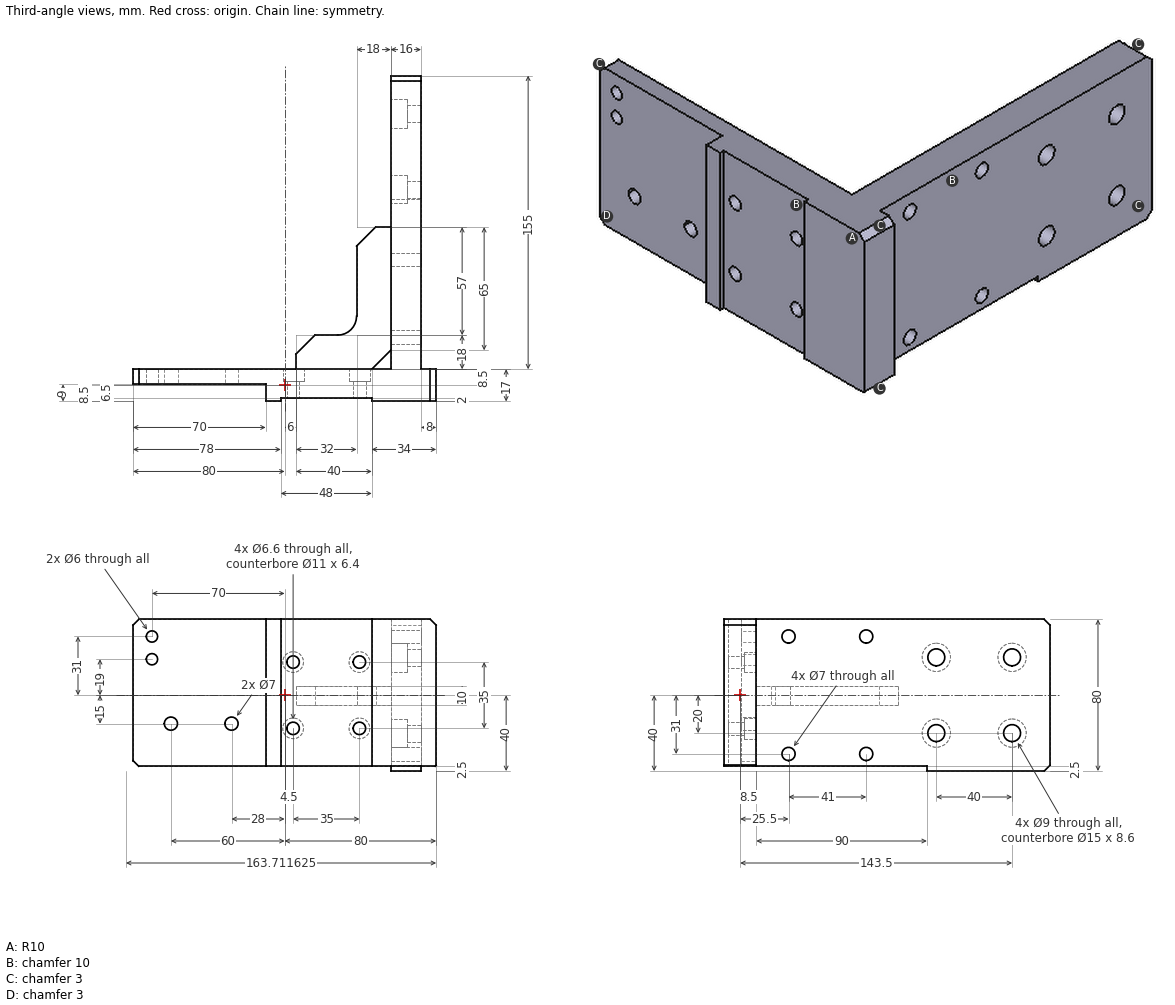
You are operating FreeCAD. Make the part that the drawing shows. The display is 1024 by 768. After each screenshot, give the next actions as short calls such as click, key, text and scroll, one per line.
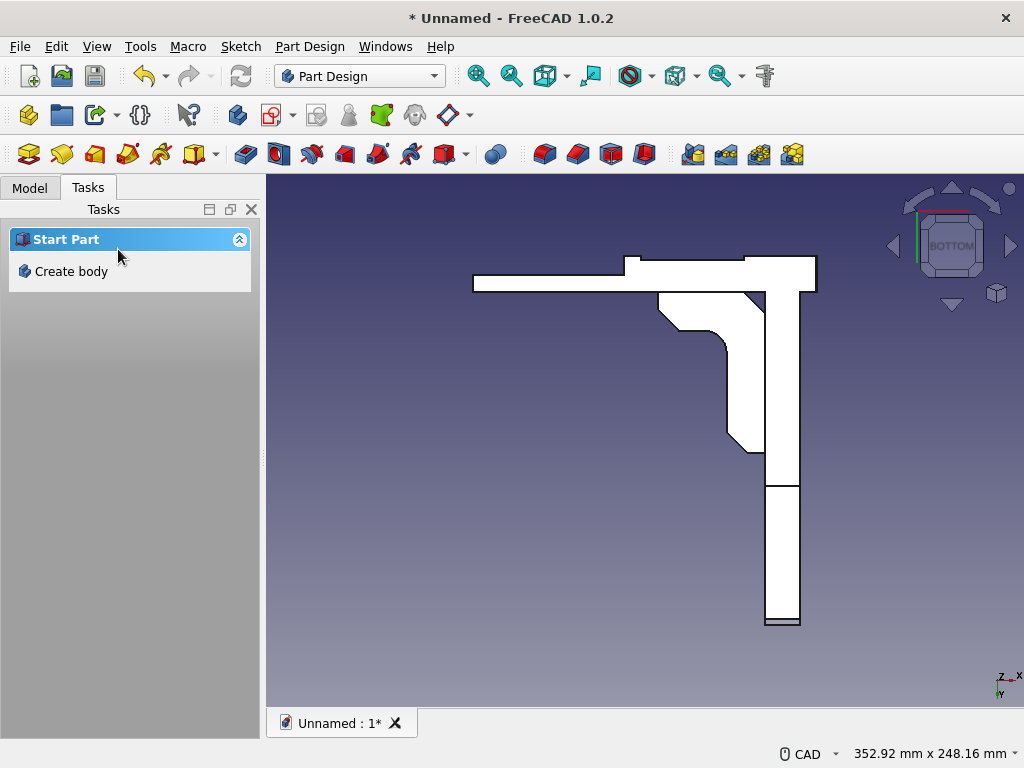
click(473, 283)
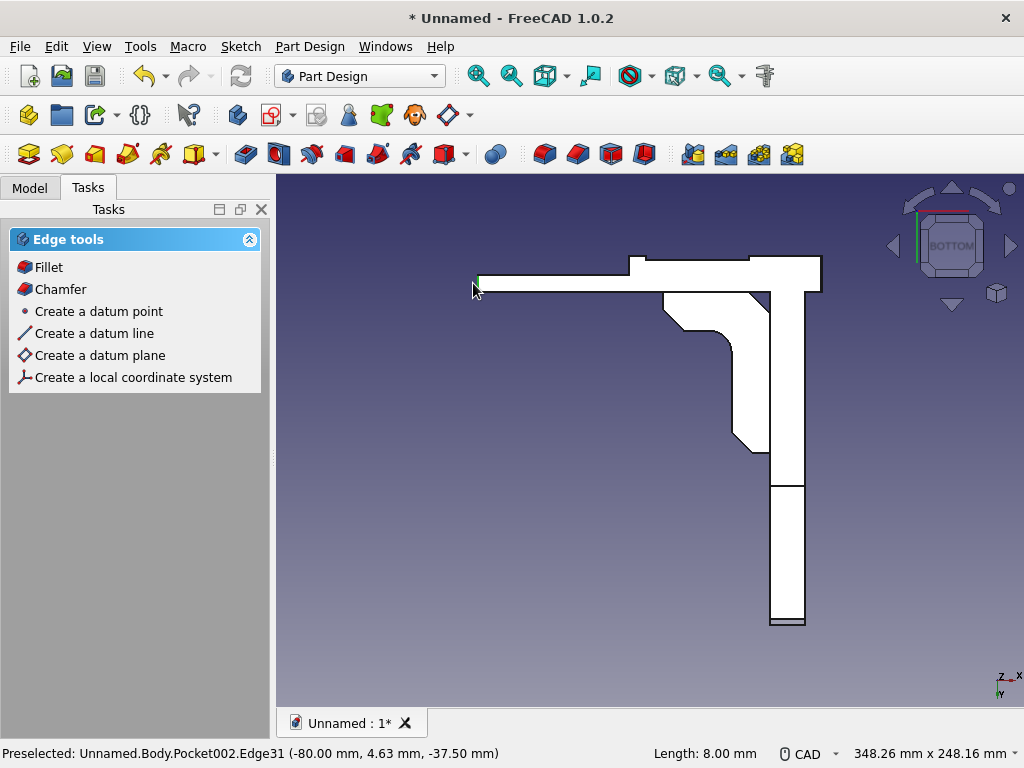
click(578, 154)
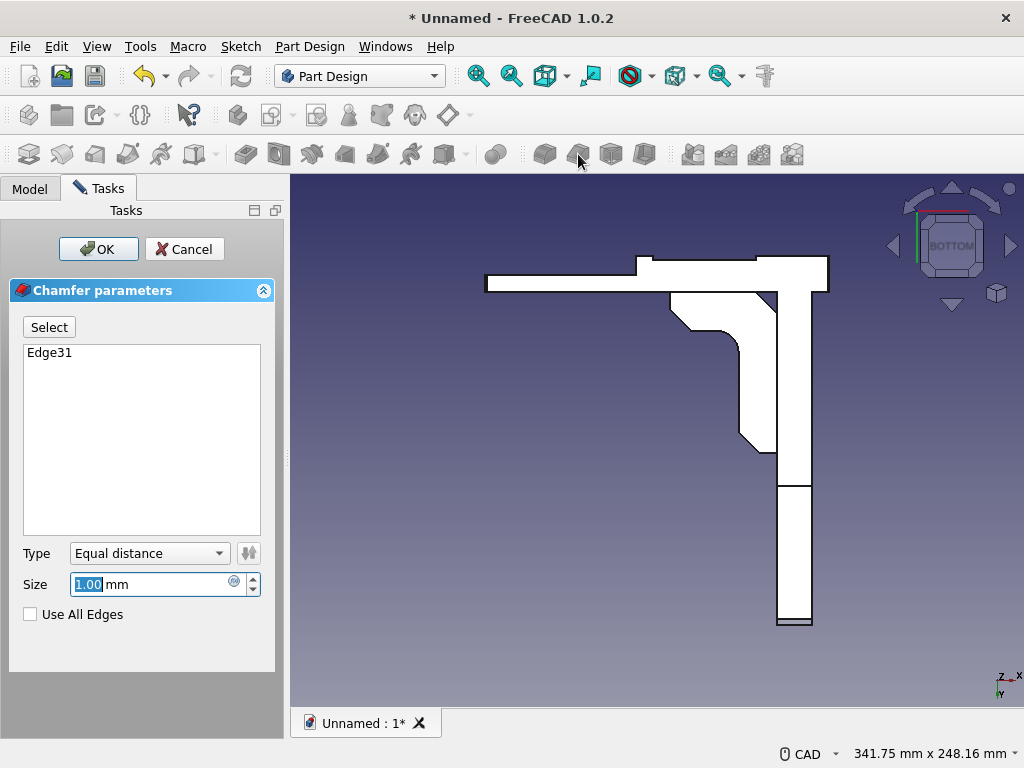
text(3)
key(Tab)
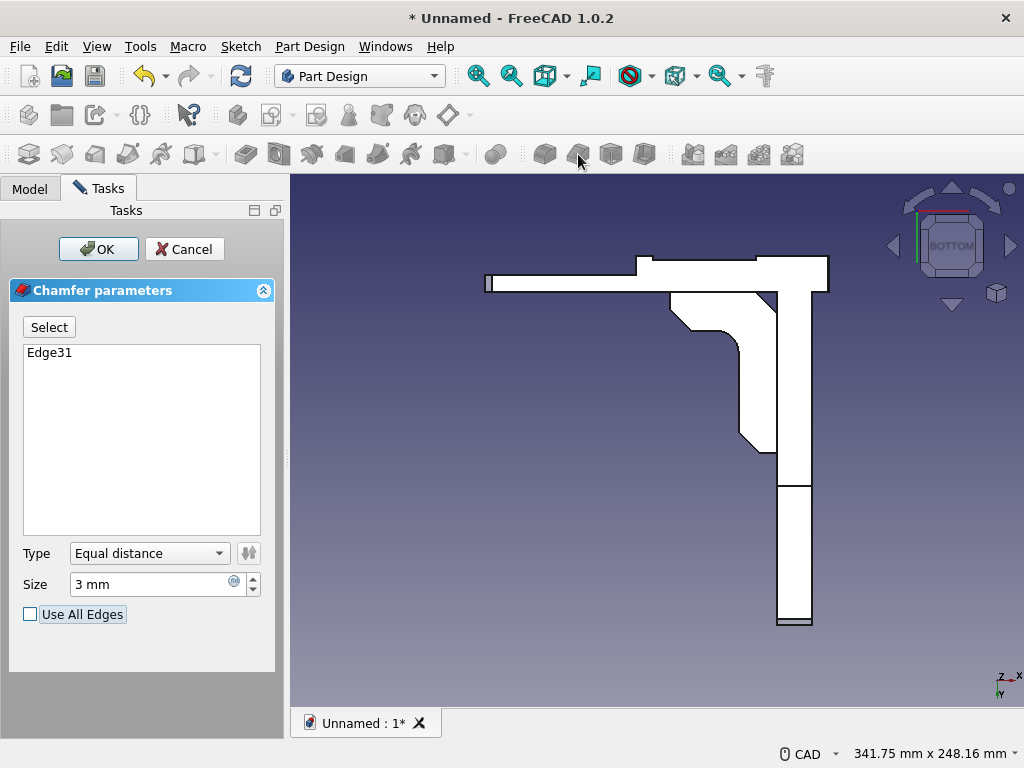
click(99, 249)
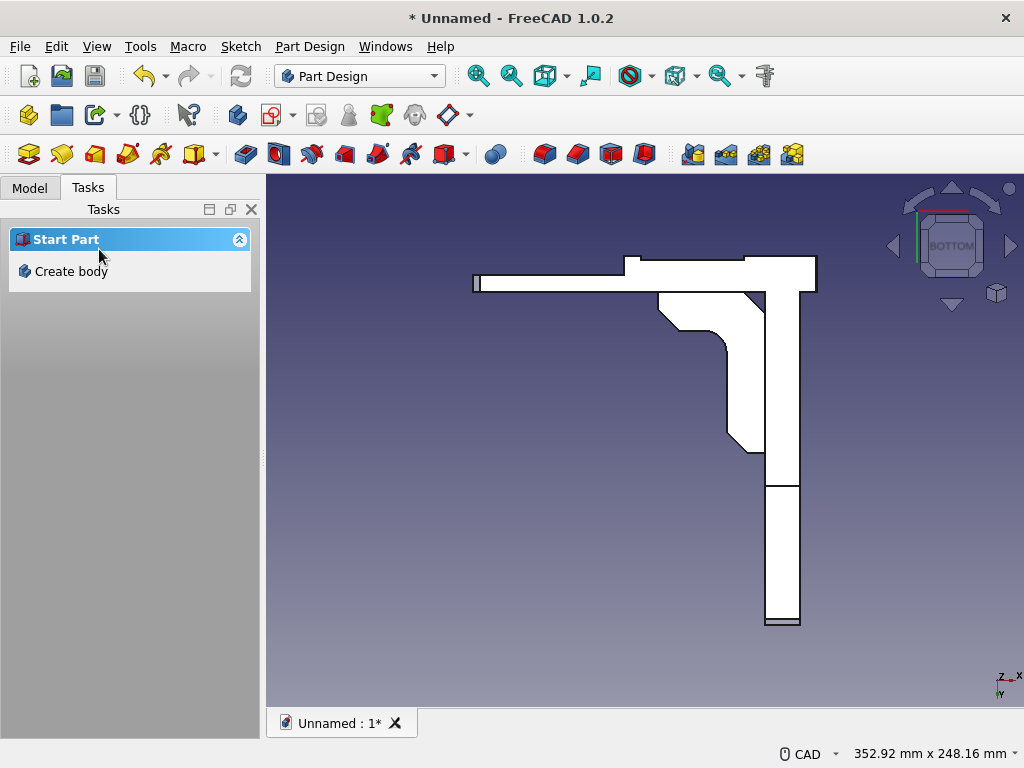
key(4)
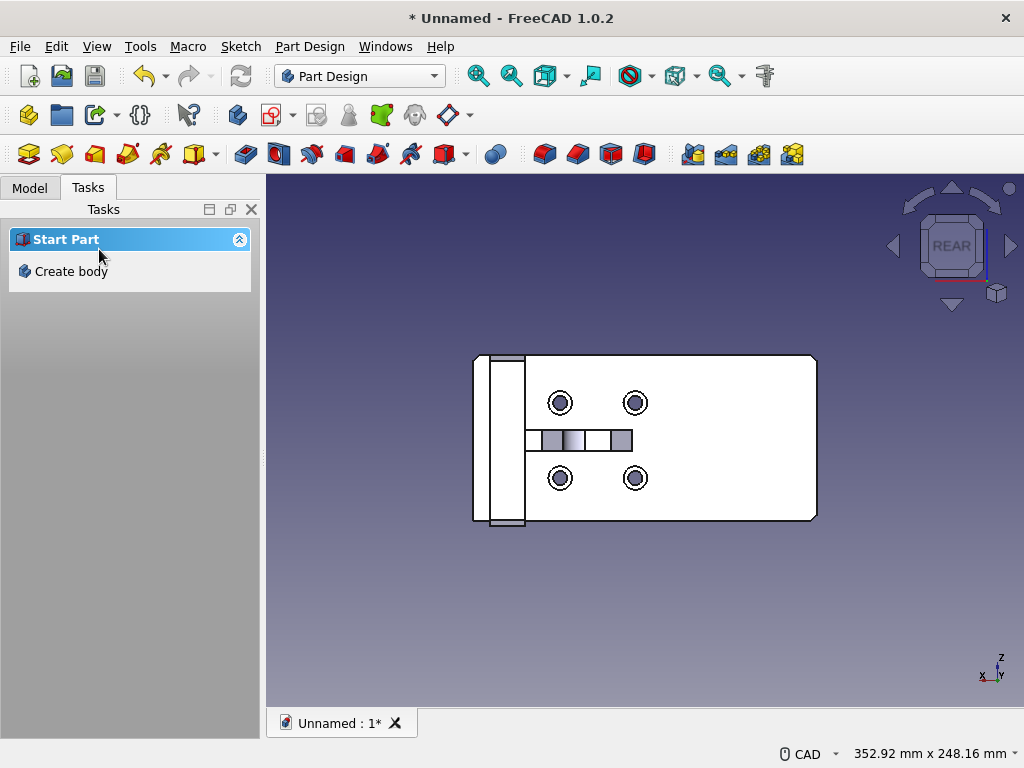
click(713, 437)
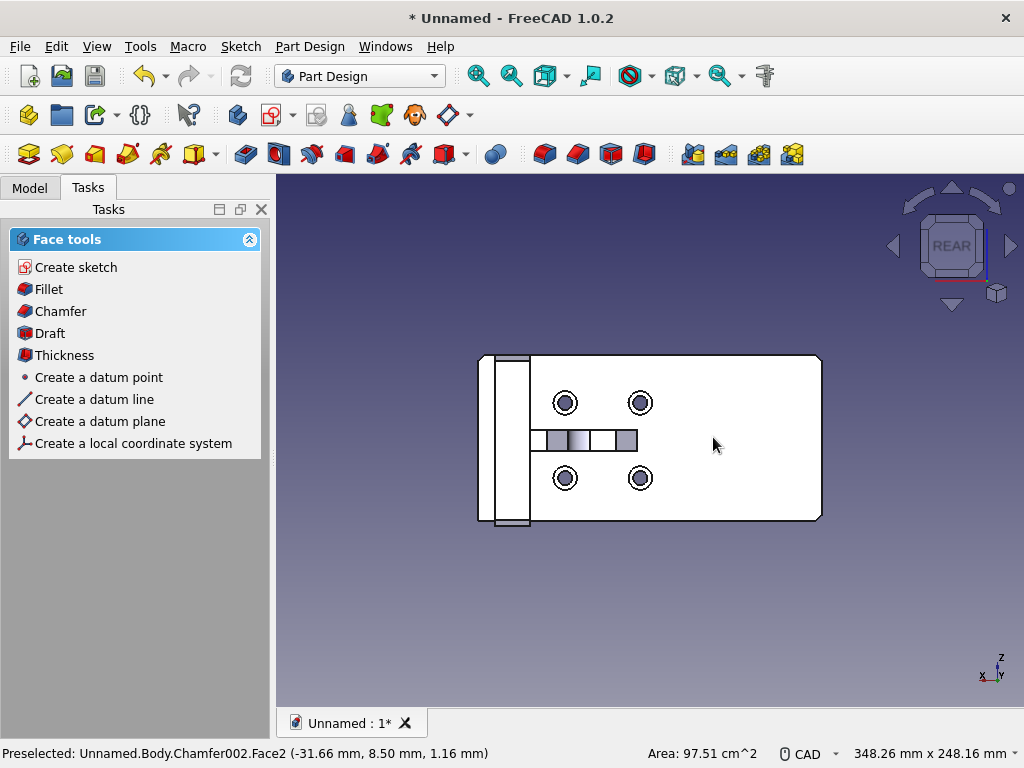
click(270, 116)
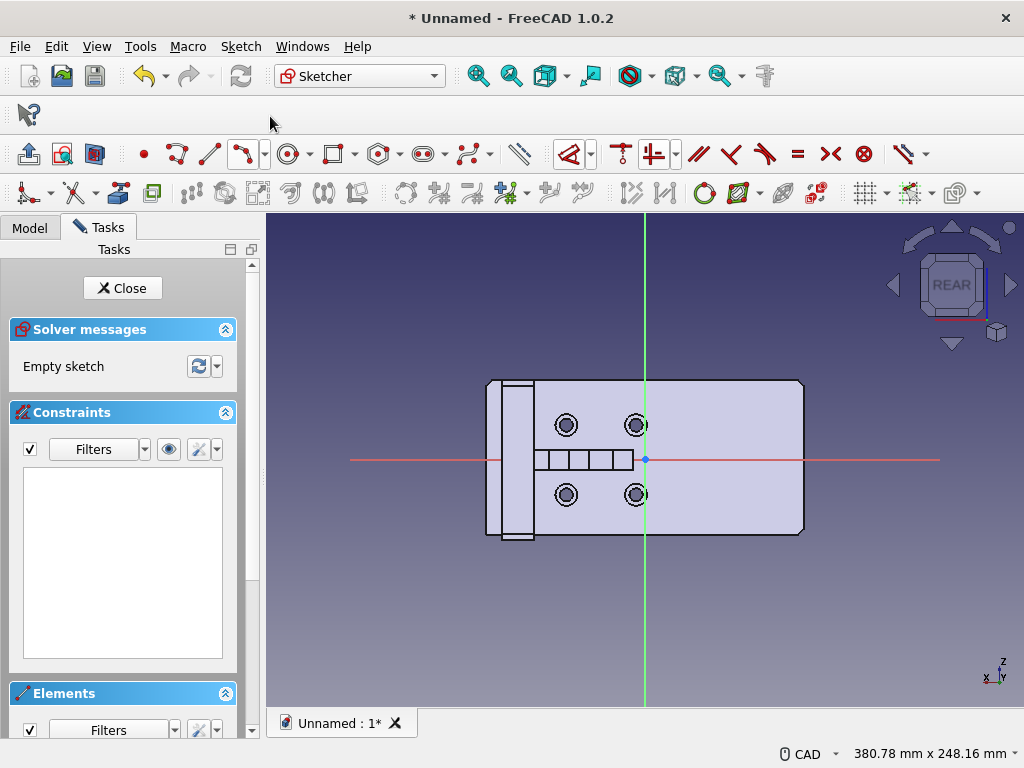
click(95, 154)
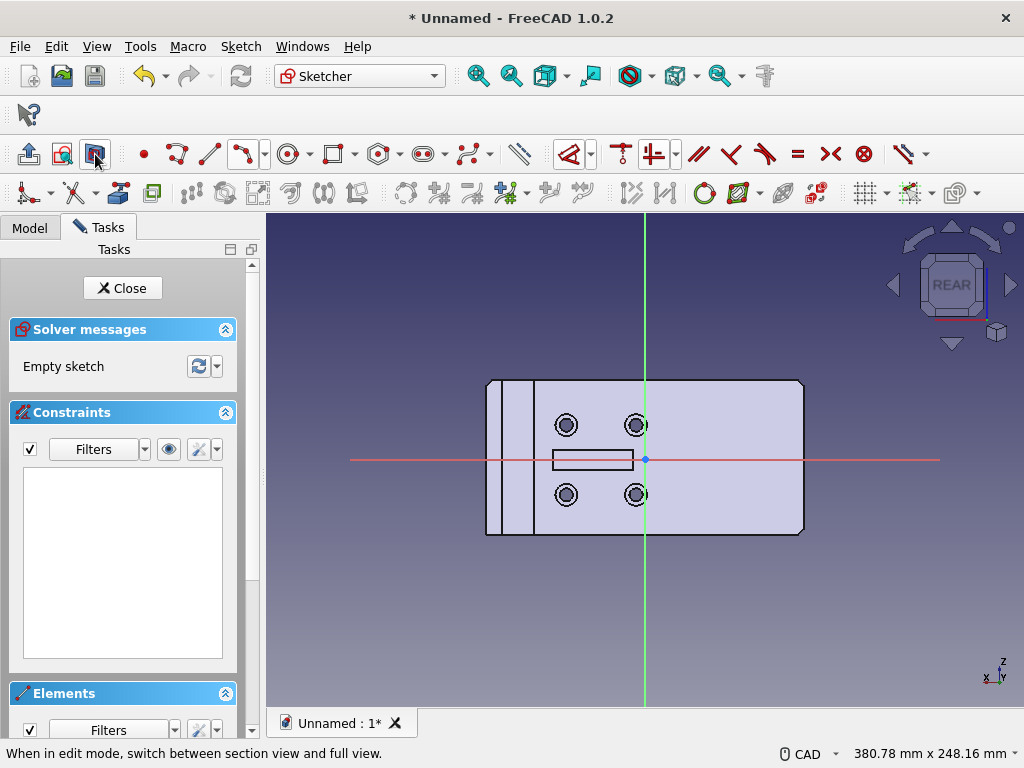
scroll(765, 486, up, 6)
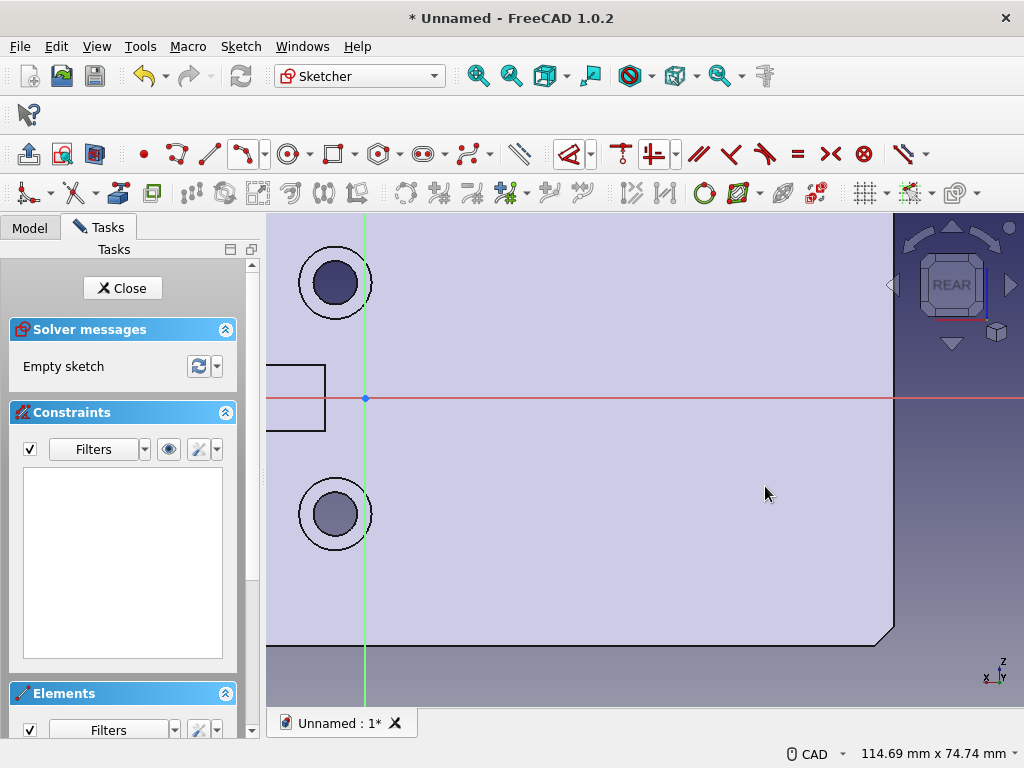
key(g)
key(c)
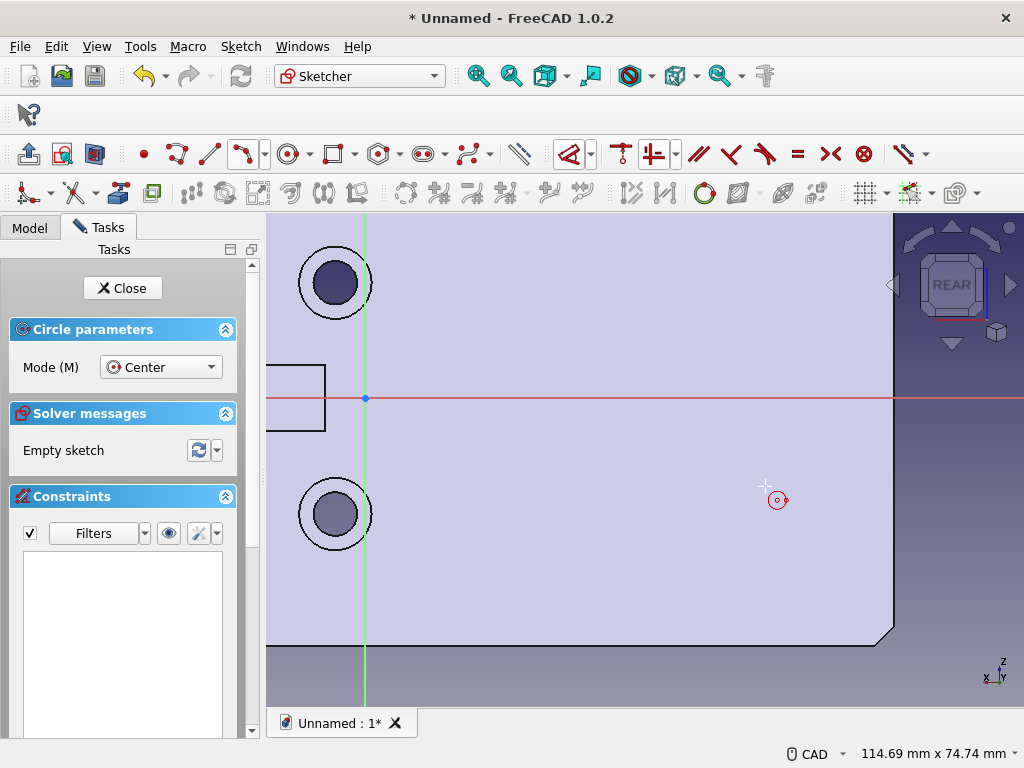
click(550, 498)
click(566, 481)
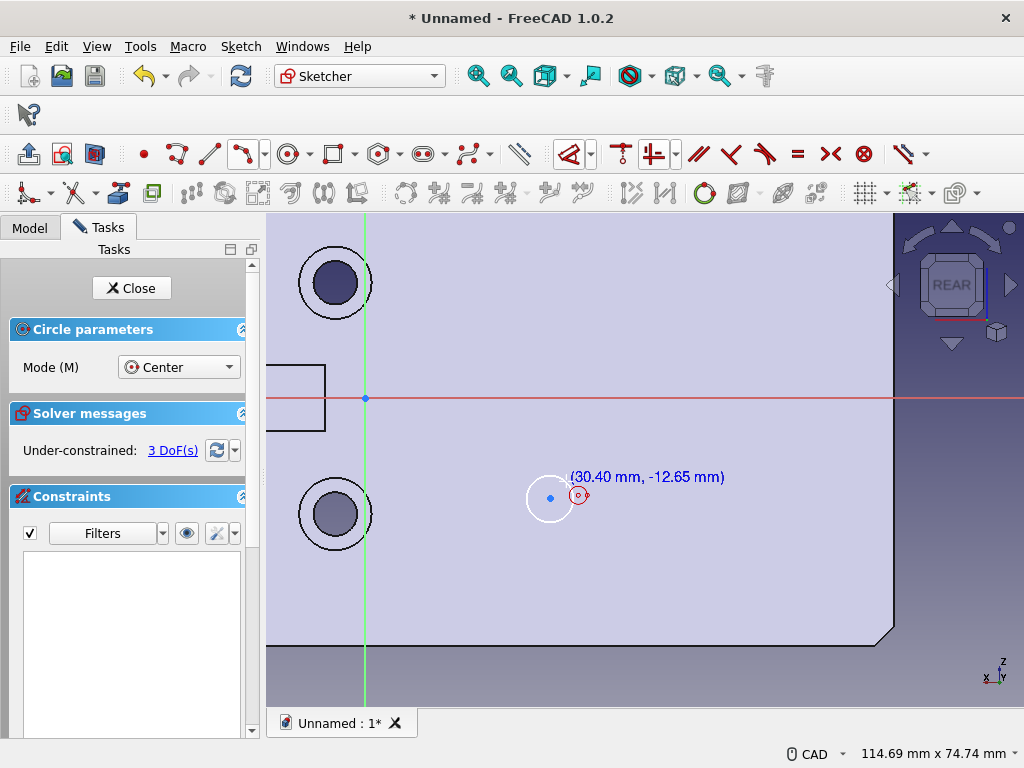
click(762, 498)
click(778, 481)
key(Escape)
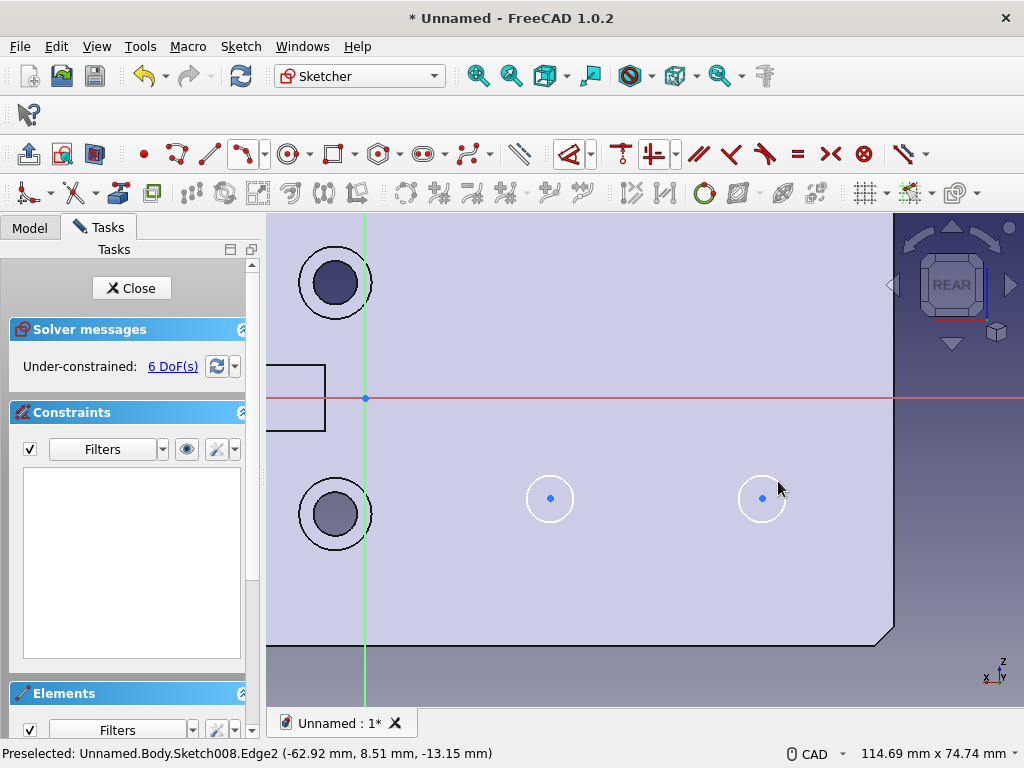
click(566, 482)